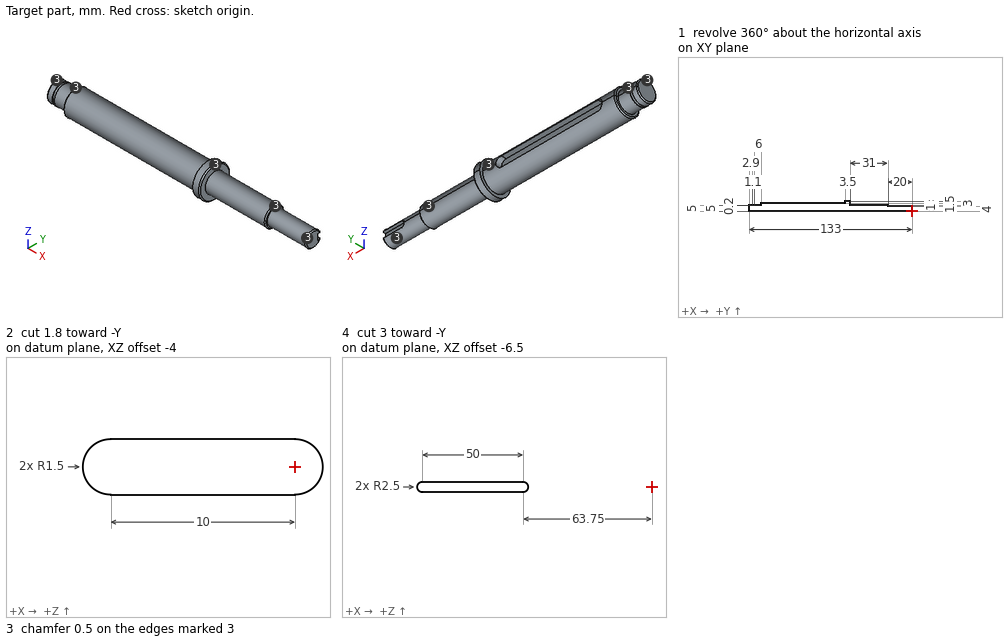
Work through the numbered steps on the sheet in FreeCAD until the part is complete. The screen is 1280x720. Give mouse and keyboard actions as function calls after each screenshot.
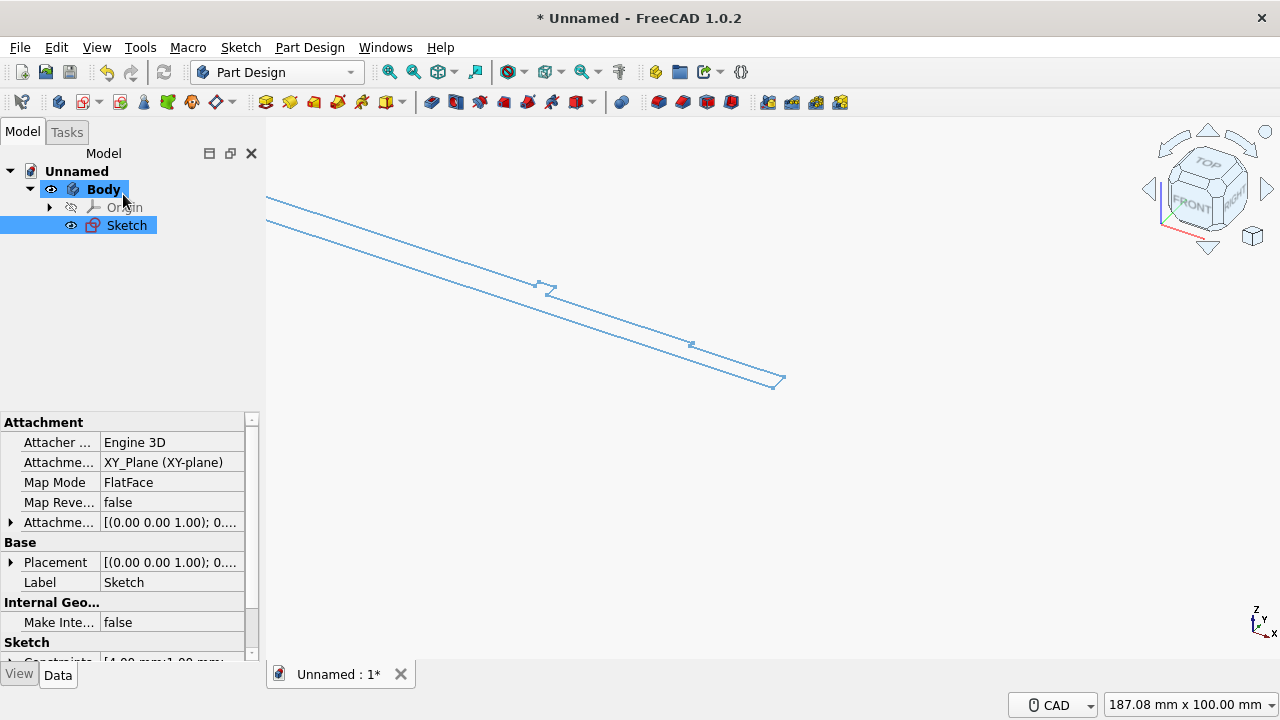
click(290, 102)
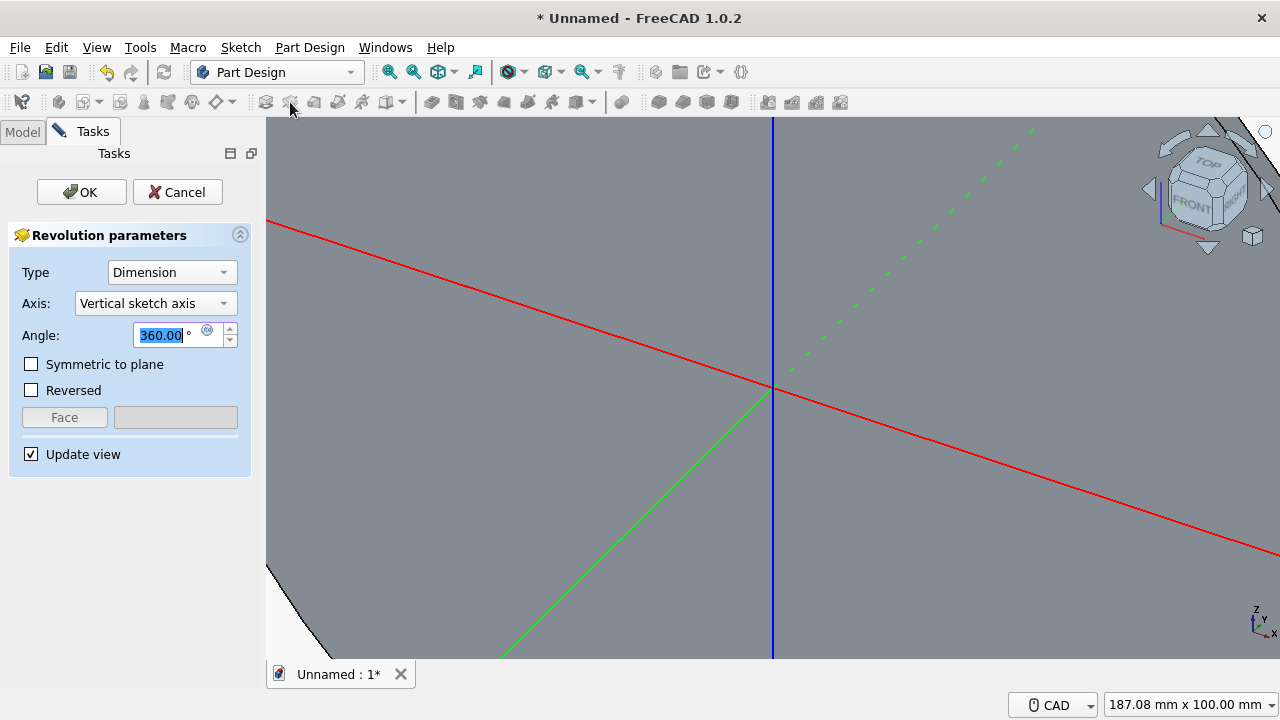
click(156, 304)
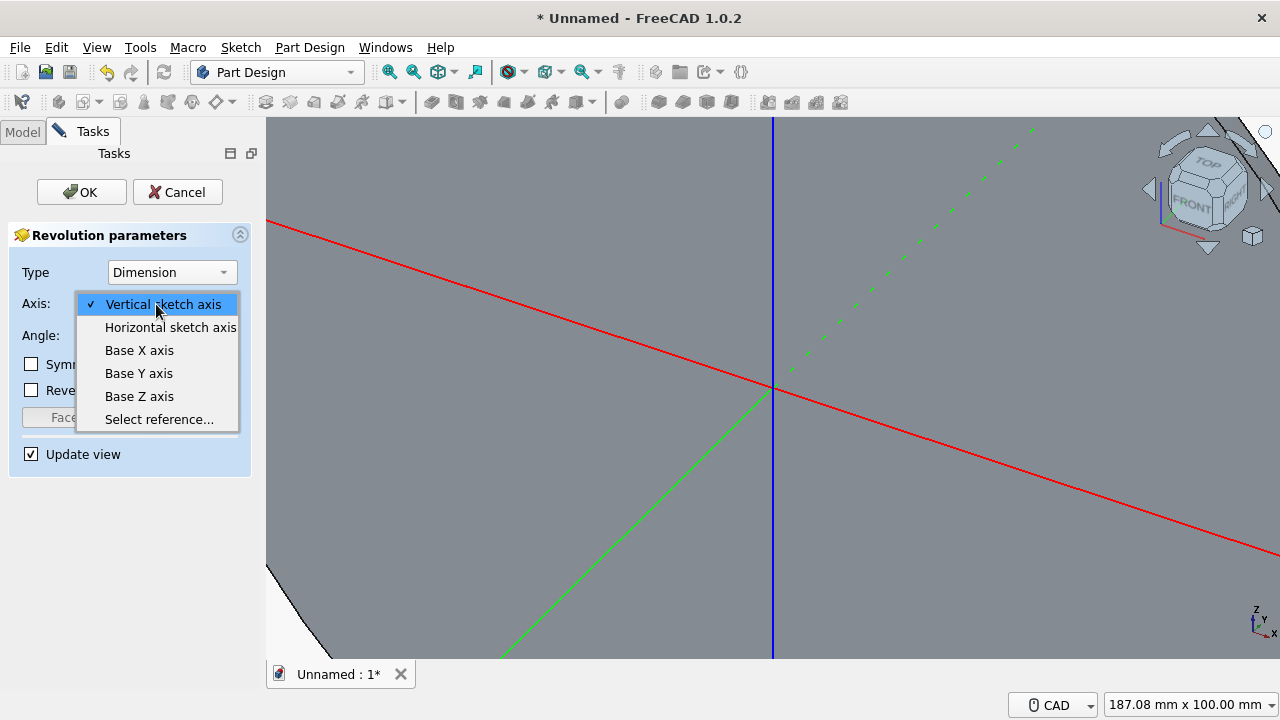
click(156, 328)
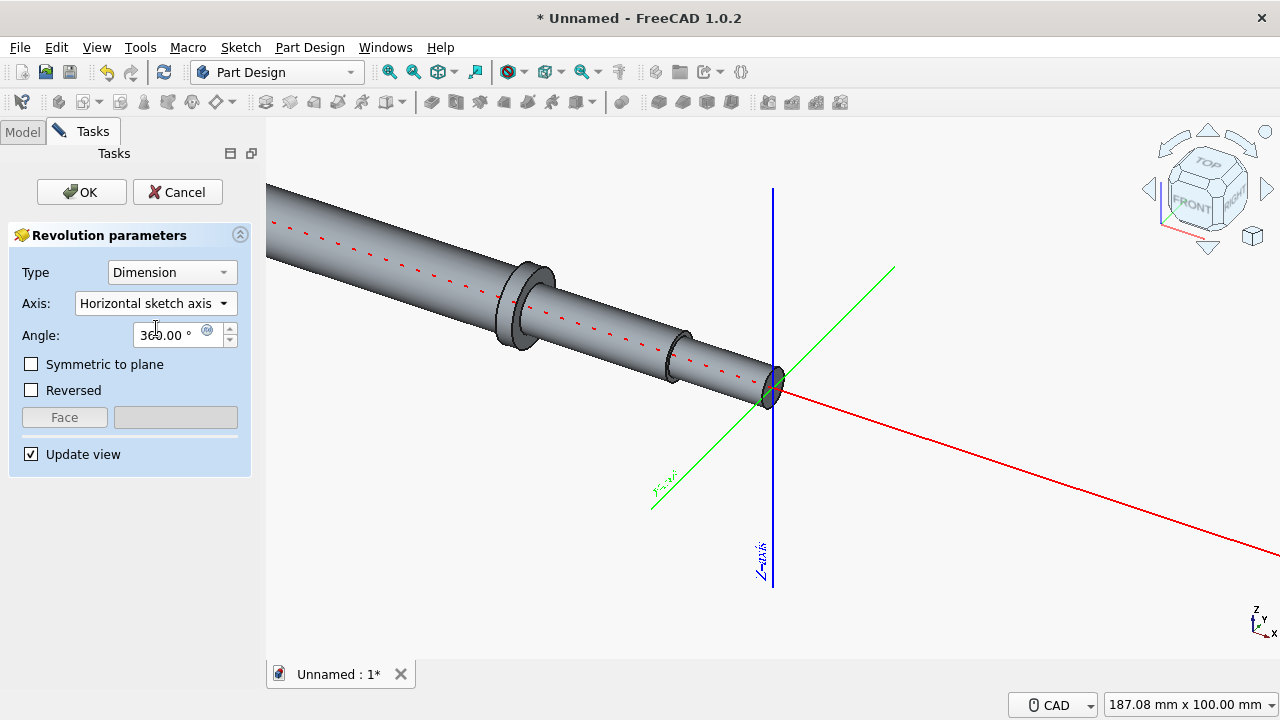
click(82, 192)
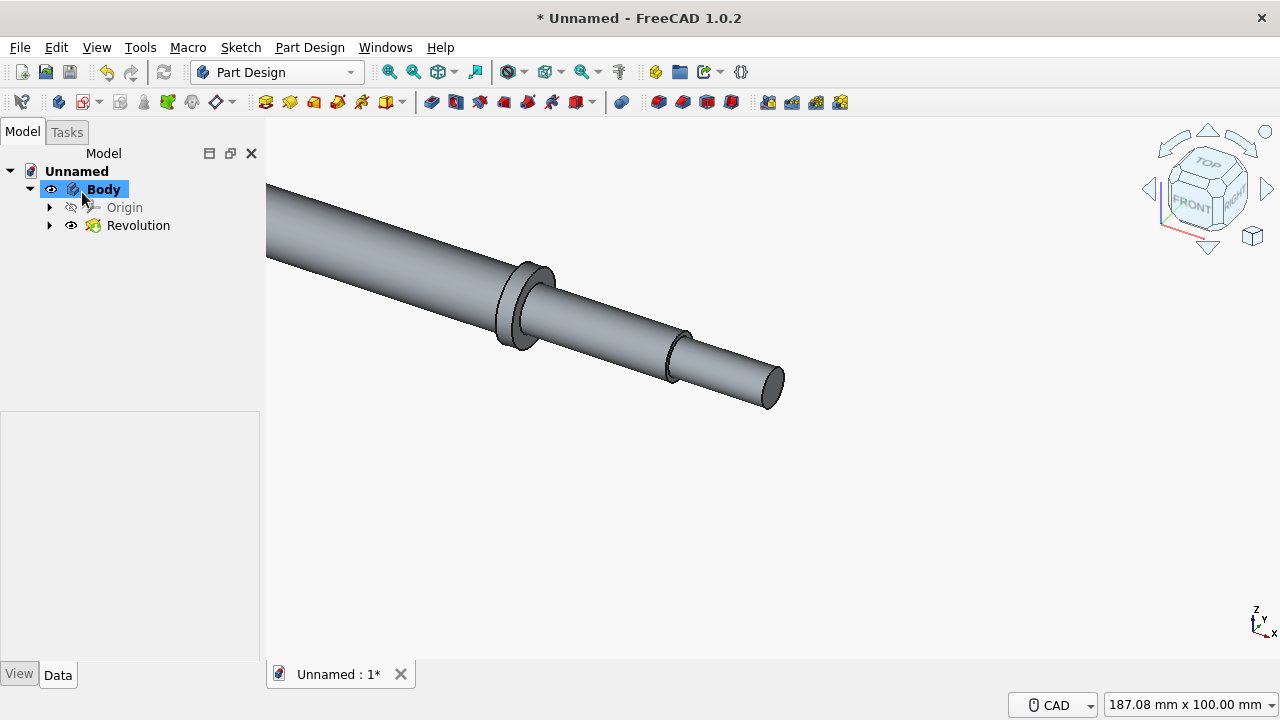
click(390, 72)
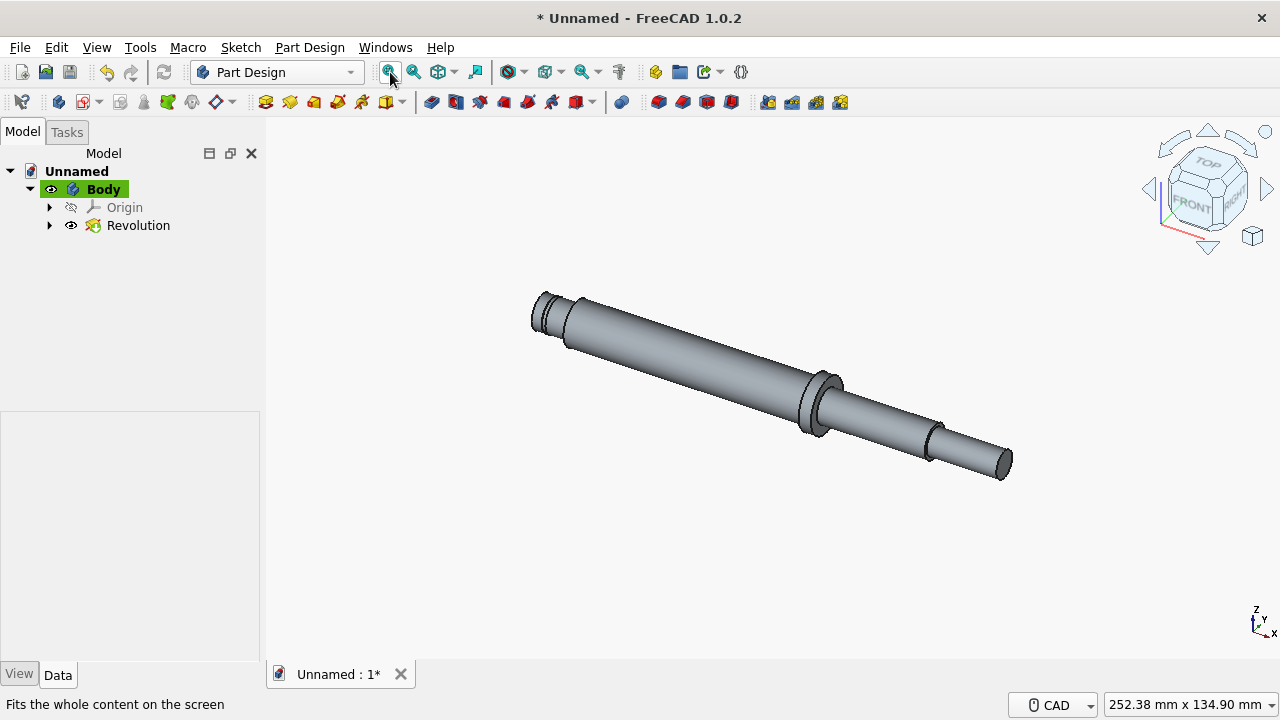
click(50, 207)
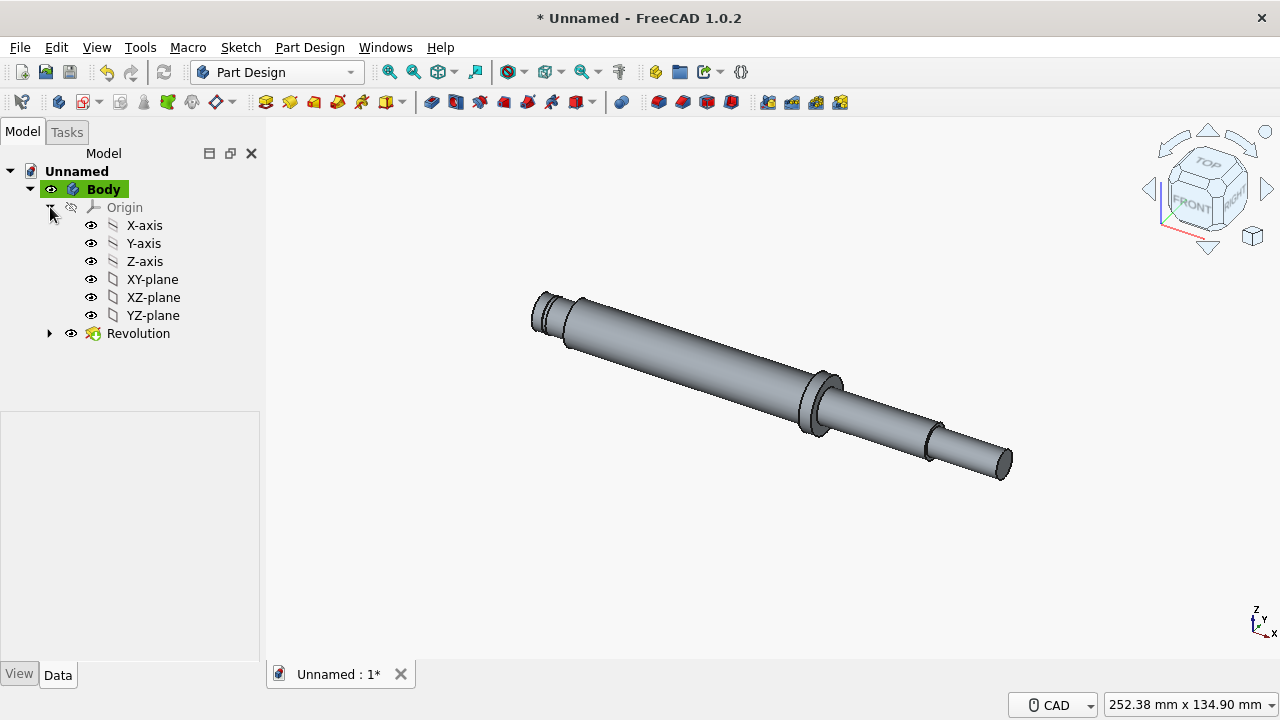
click(136, 297)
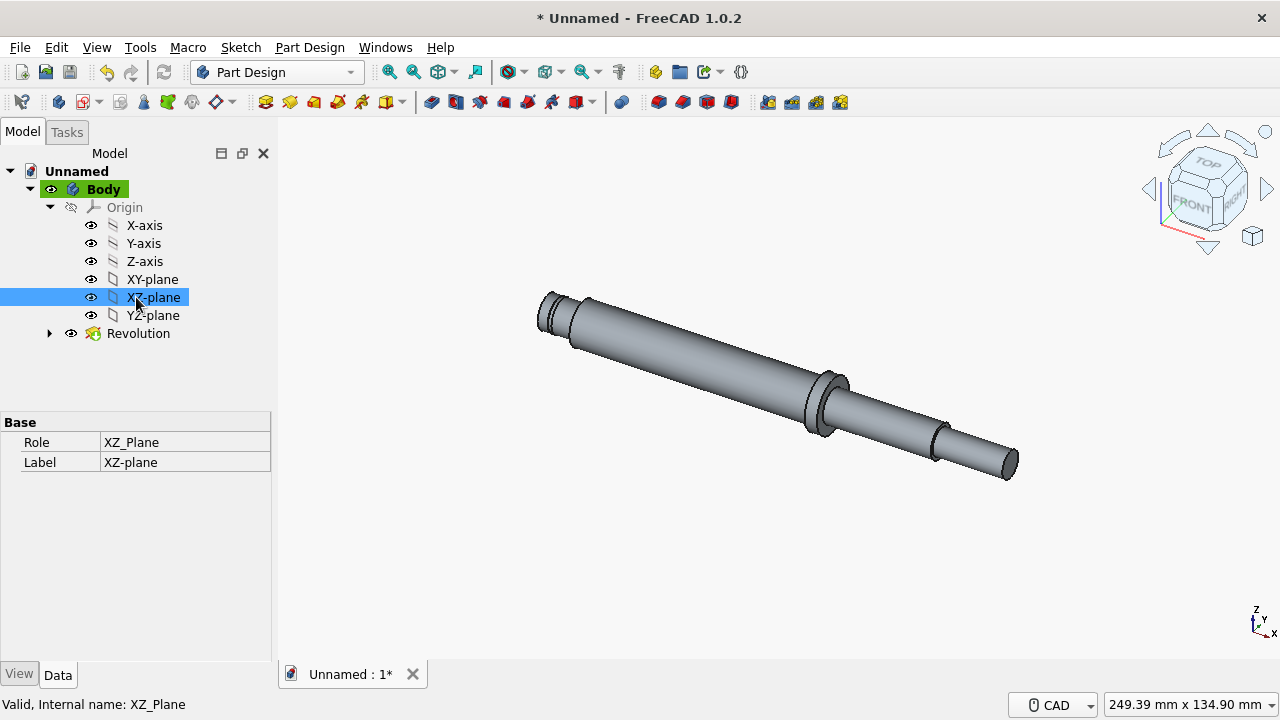
click(216, 102)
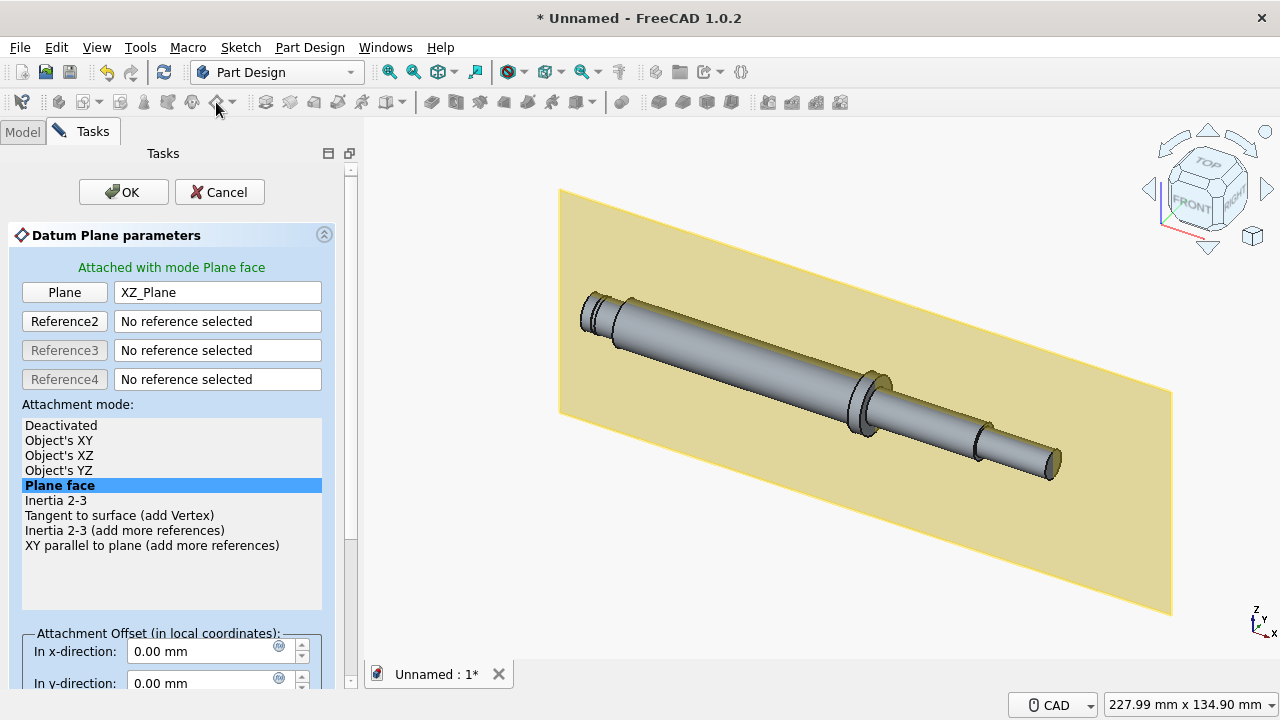
scroll(351, 426, down, 2)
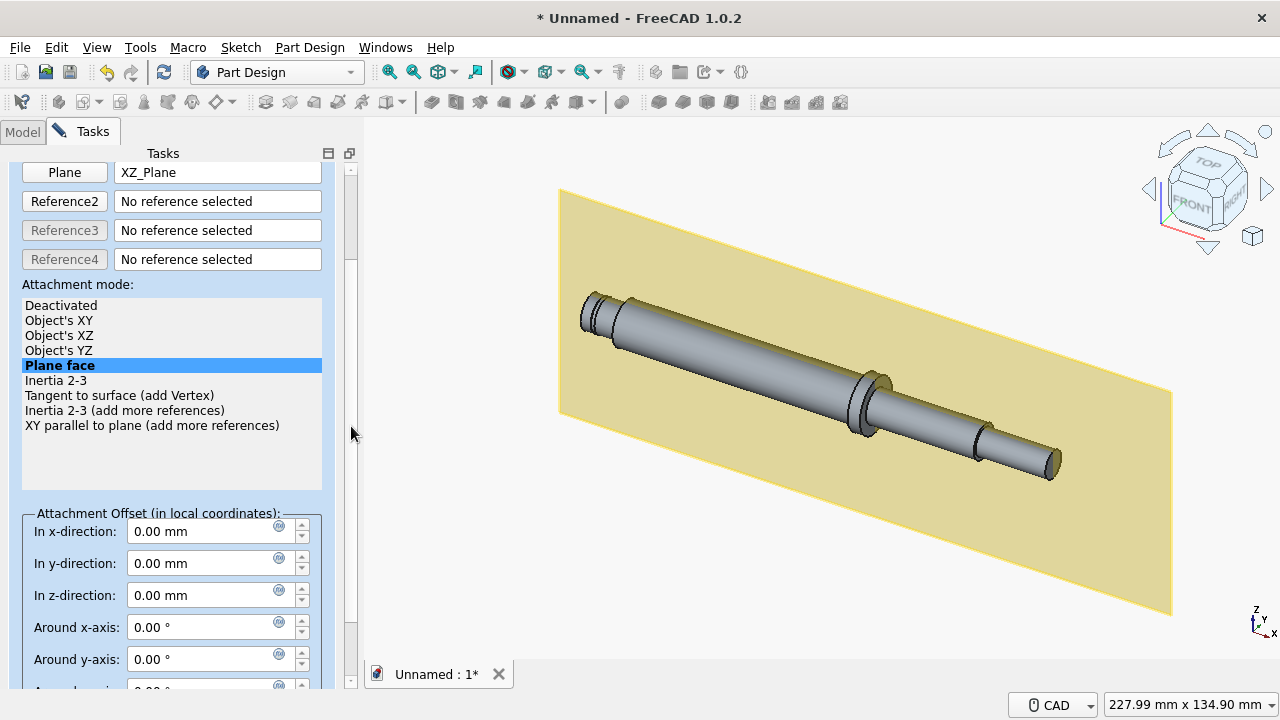
triple_click(210, 595)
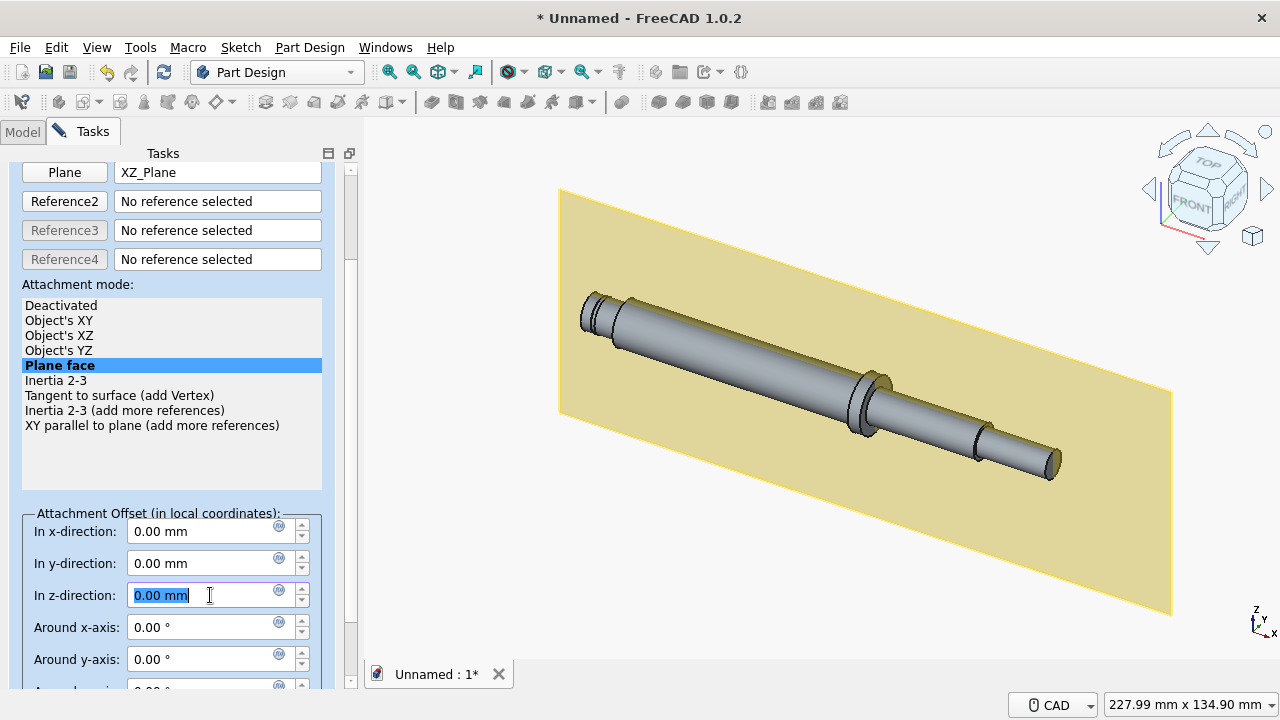
text(-4)
key(Tab)